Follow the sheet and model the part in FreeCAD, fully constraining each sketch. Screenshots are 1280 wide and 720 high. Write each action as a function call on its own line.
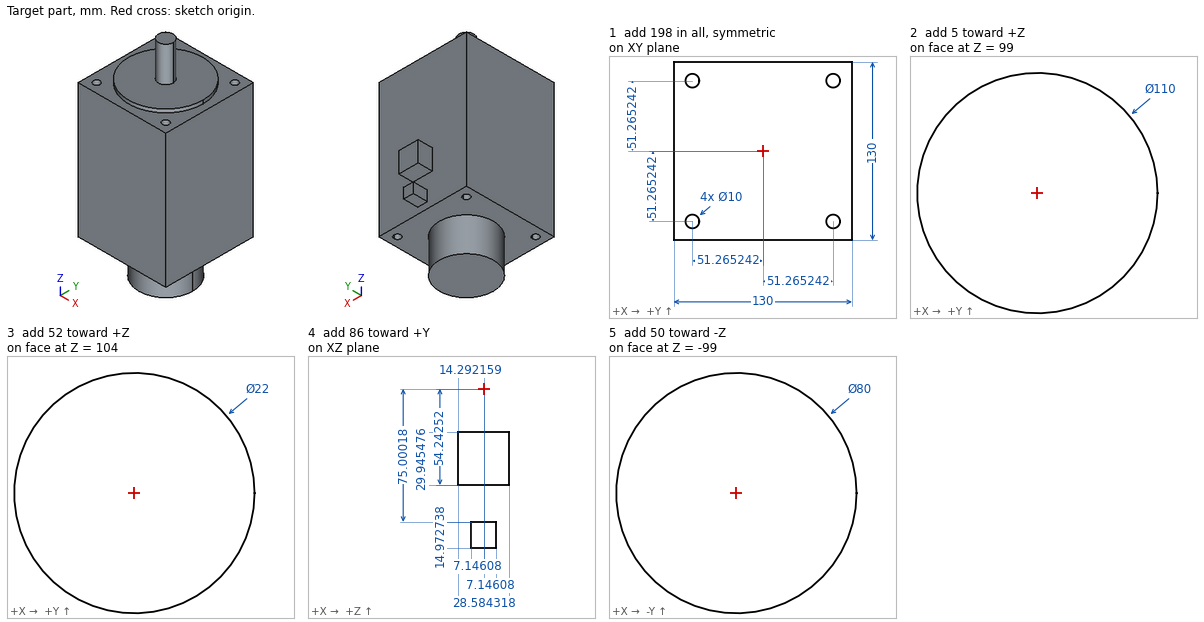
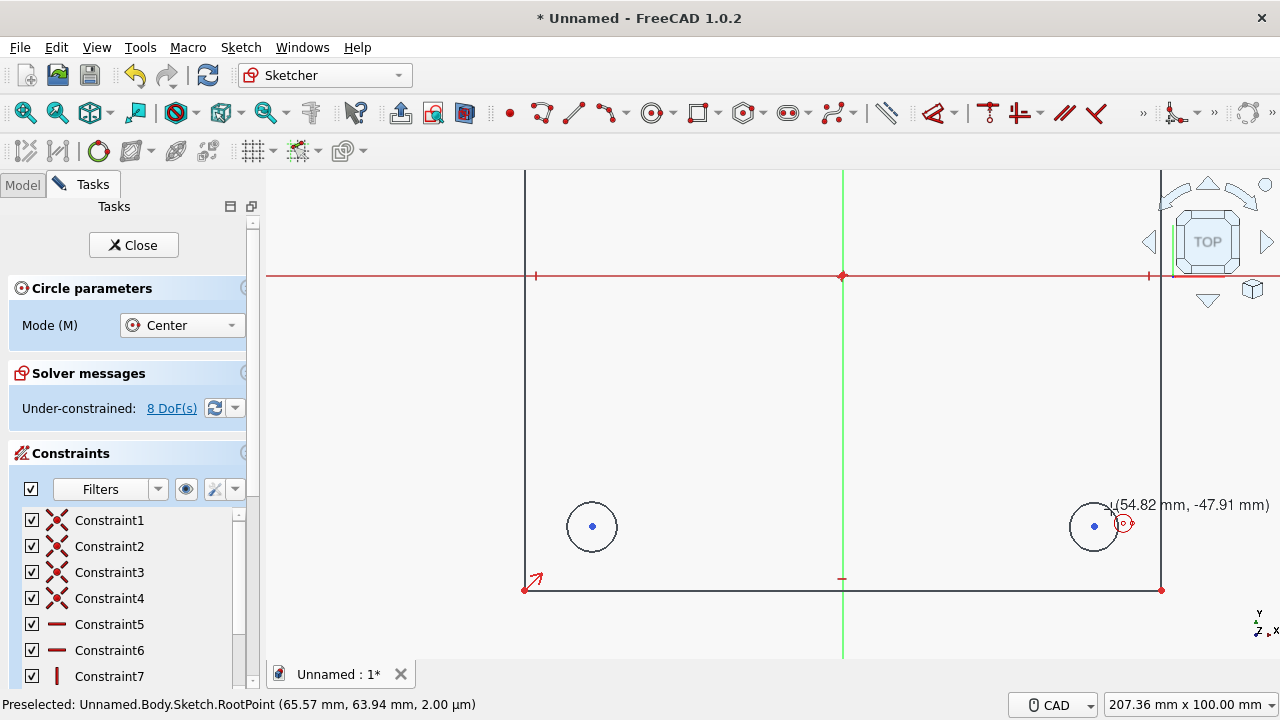
scroll(592, 528, down, 4)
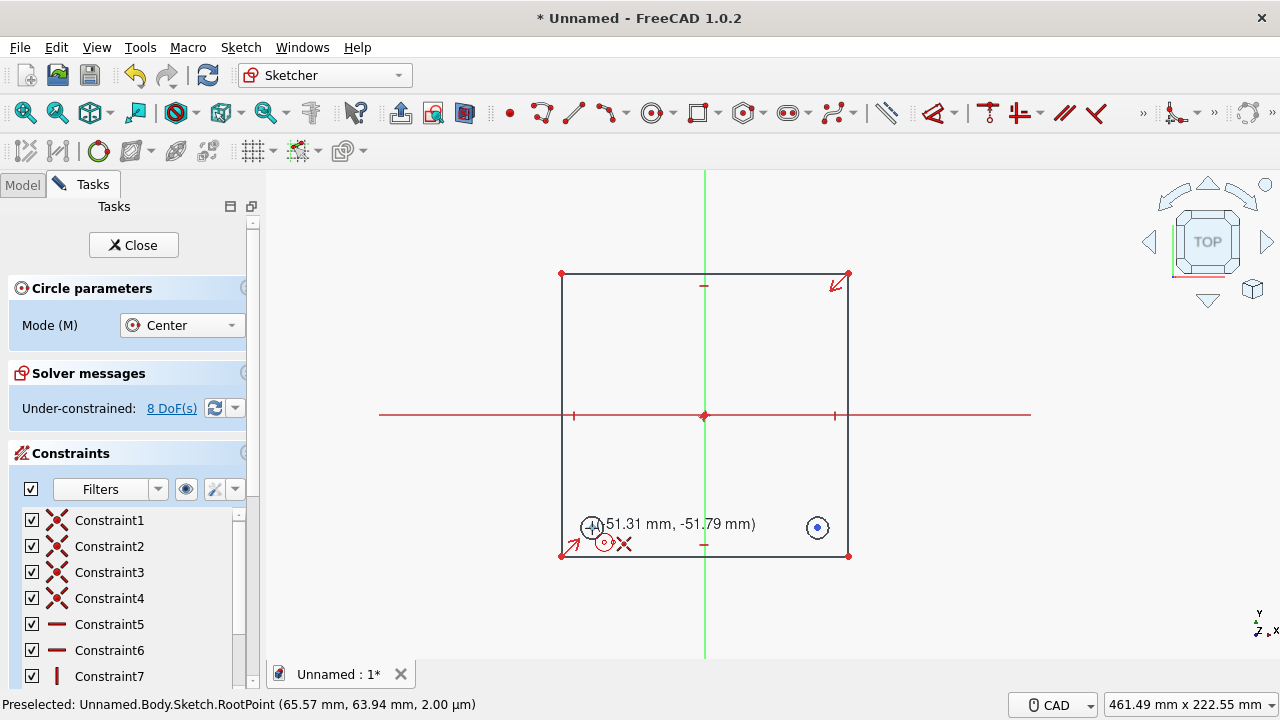
scroll(592, 302, up, 4)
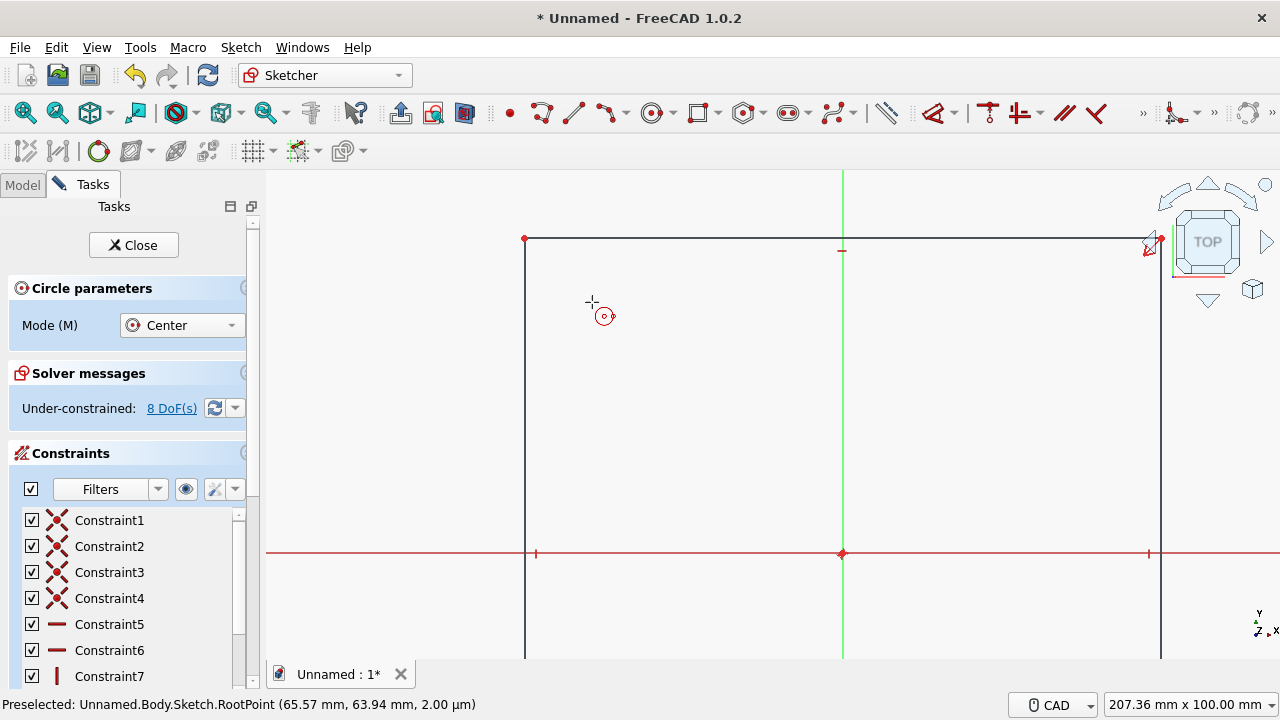
click(592, 303)
click(610, 285)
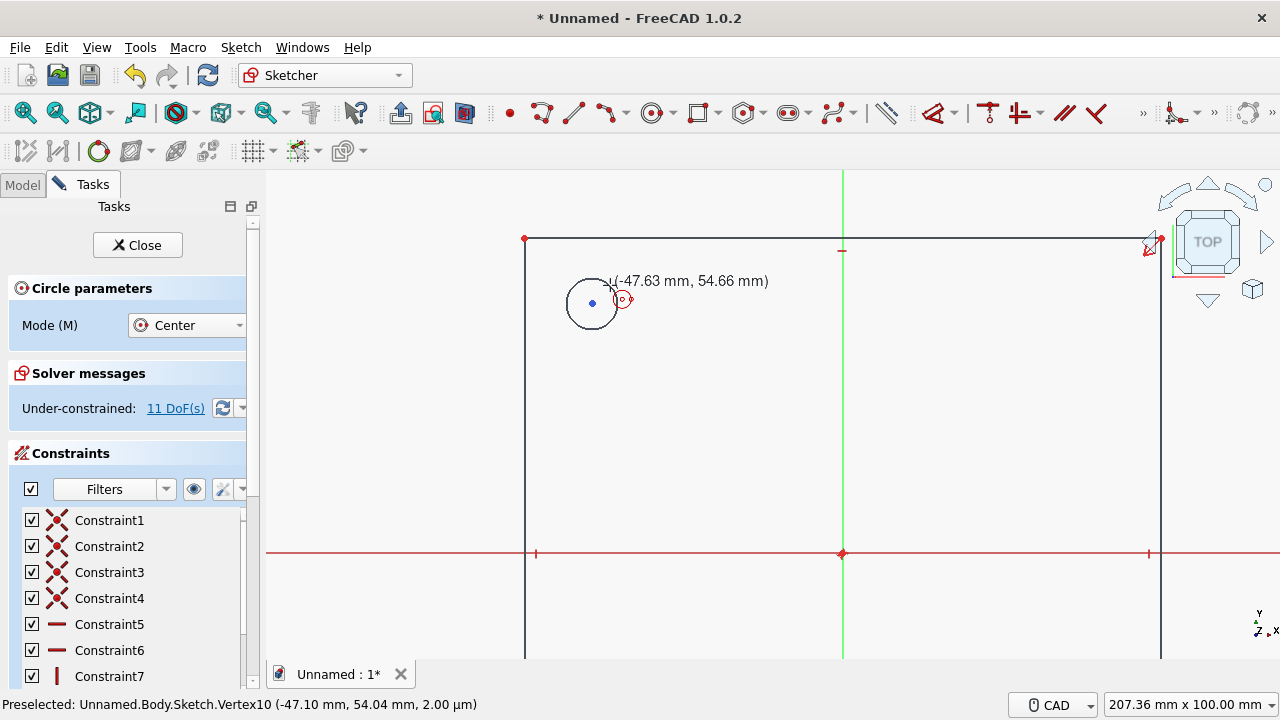
click(1094, 303)
click(1111, 285)
key(Escape)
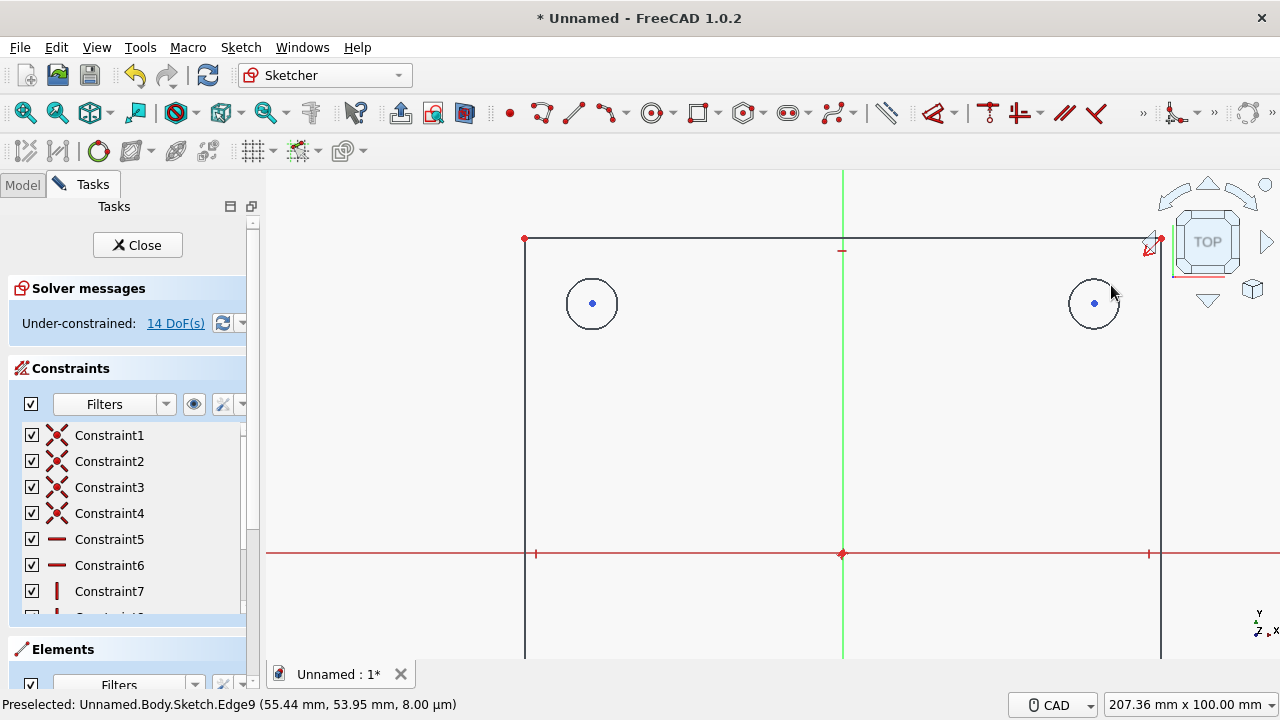
scroll(592, 301, down, 4)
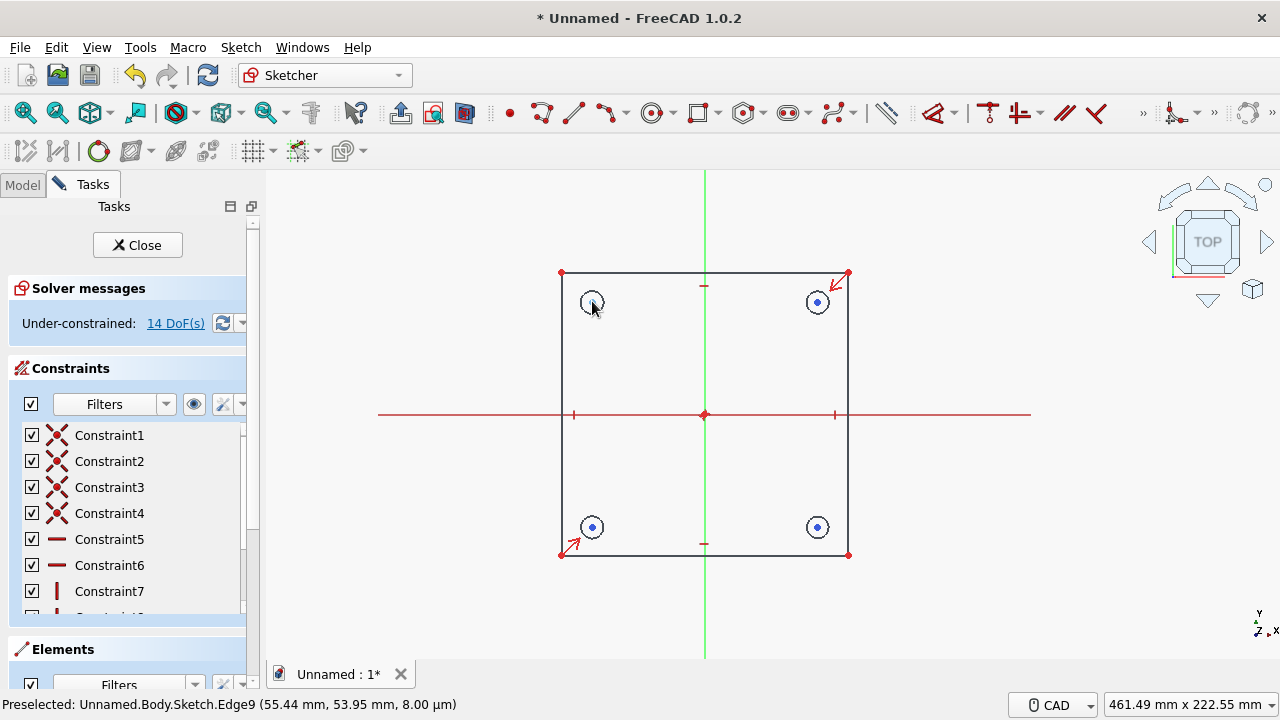
scroll(600, 520, up, 2)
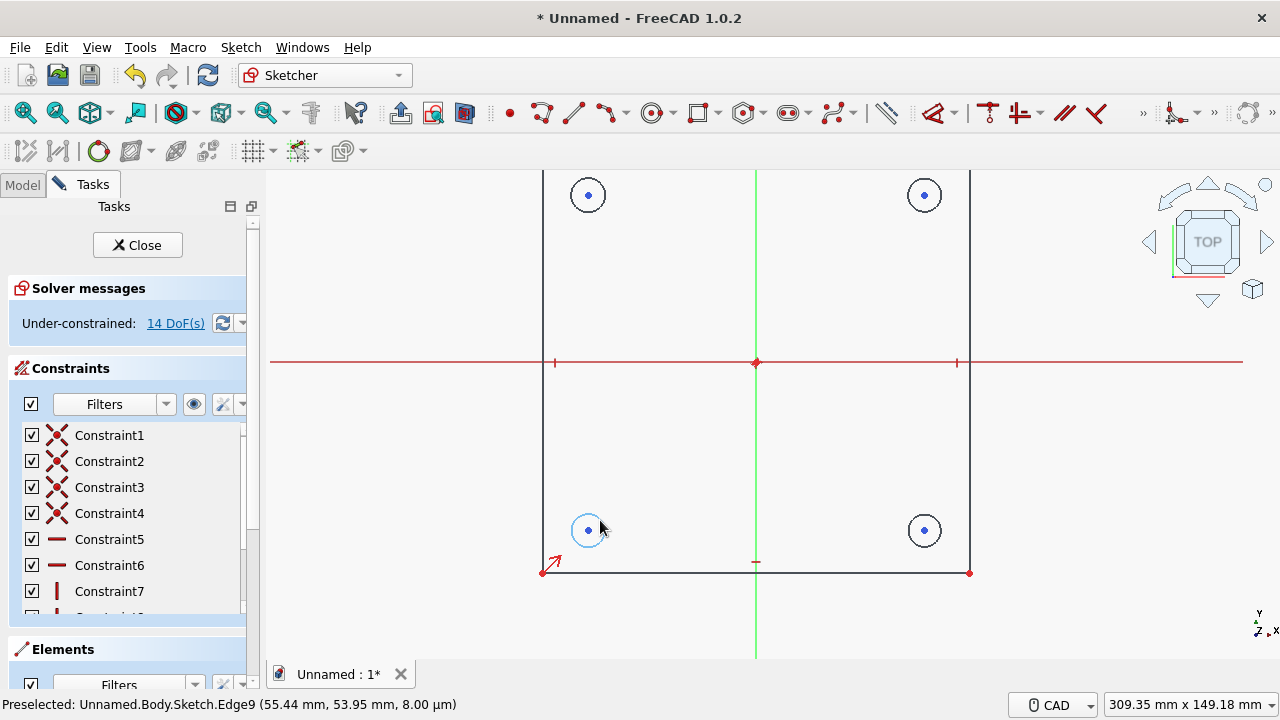
click(600, 519)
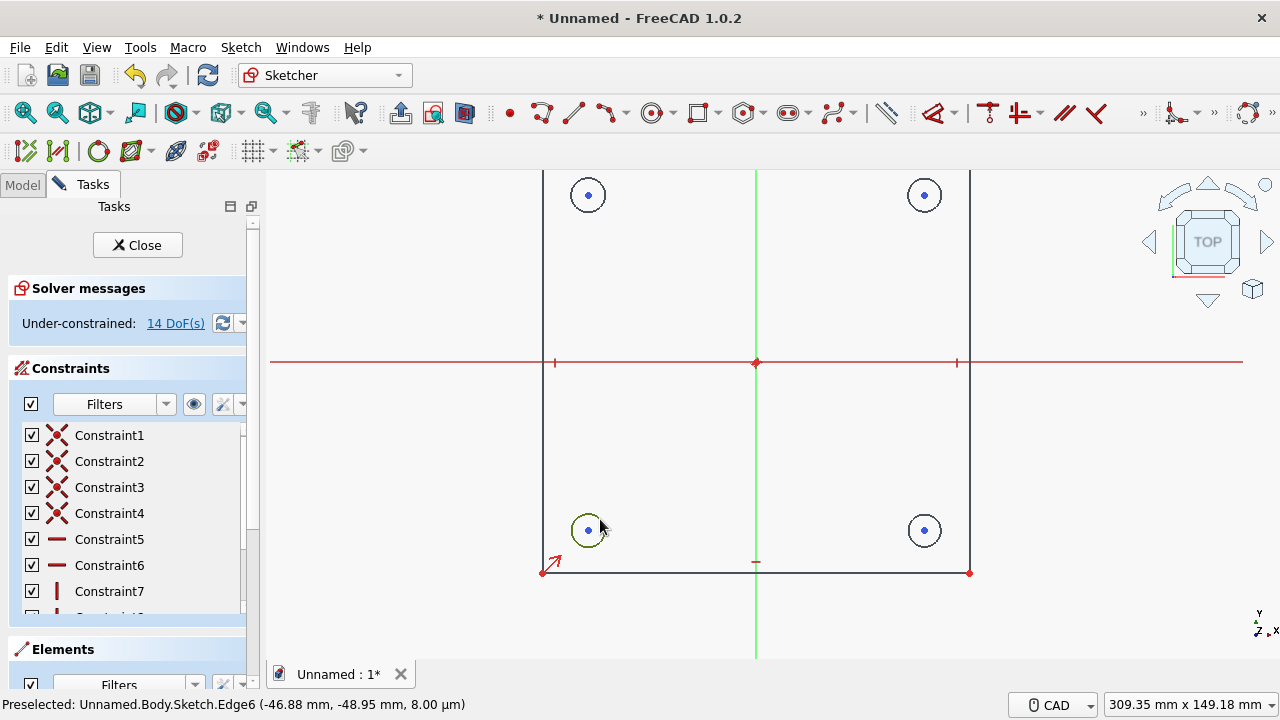
click(936, 519)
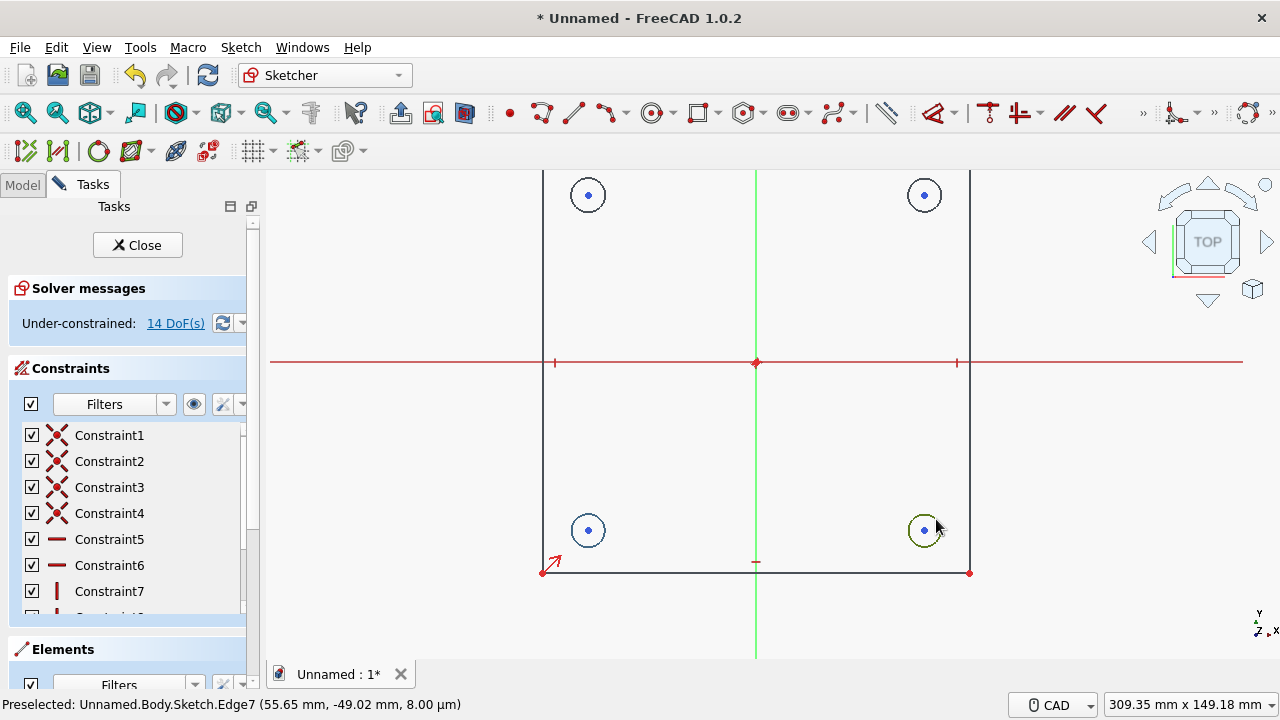
click(576, 207)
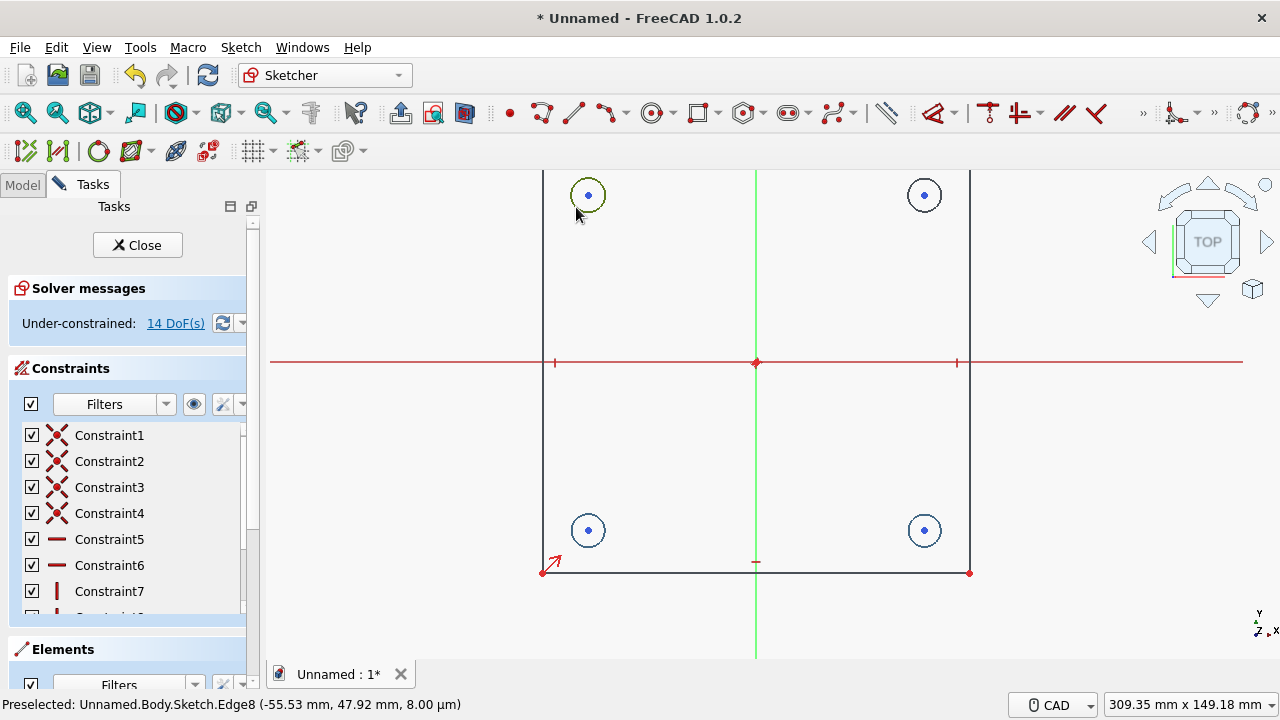
click(913, 207)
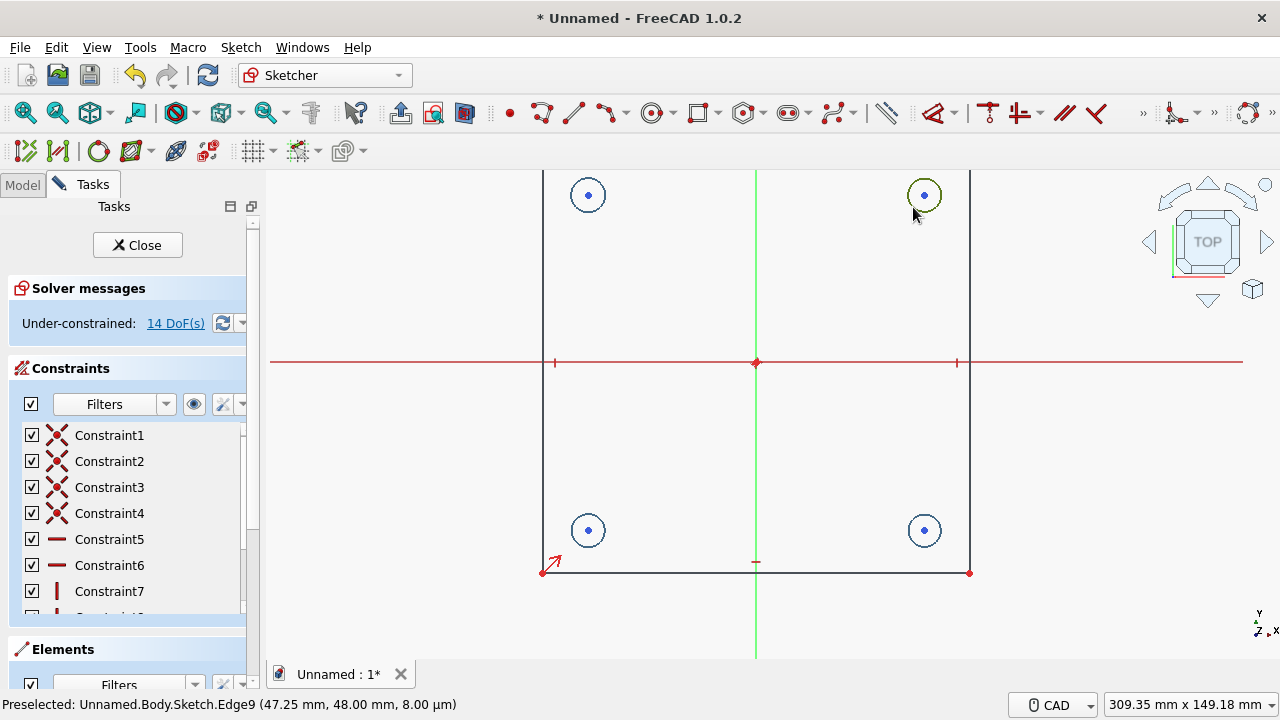
key(e)